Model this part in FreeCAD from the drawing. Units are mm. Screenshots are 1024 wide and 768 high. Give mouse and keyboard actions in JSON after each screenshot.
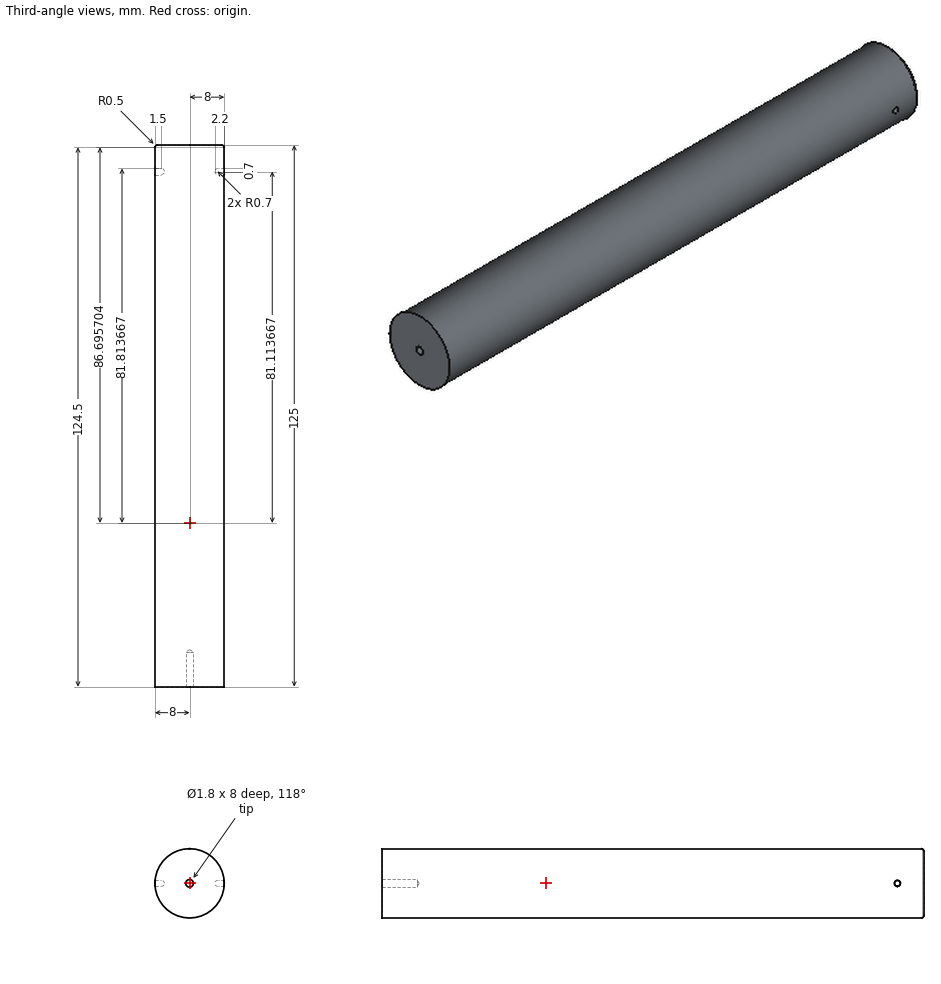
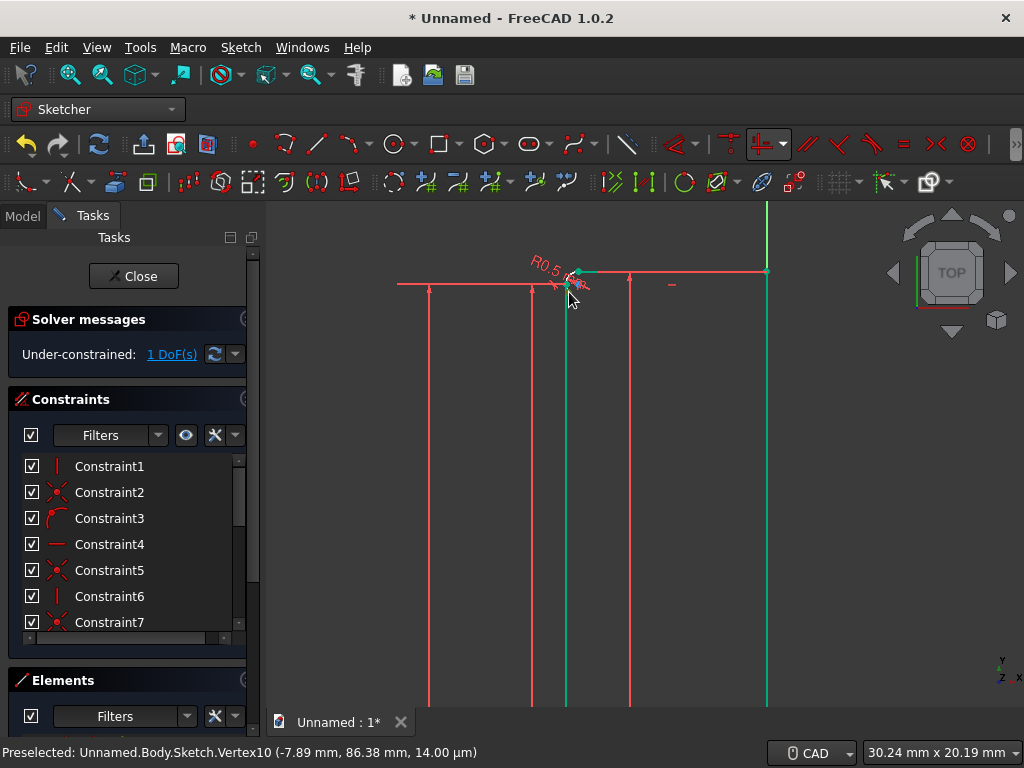
{"action": "key", "text": "i"}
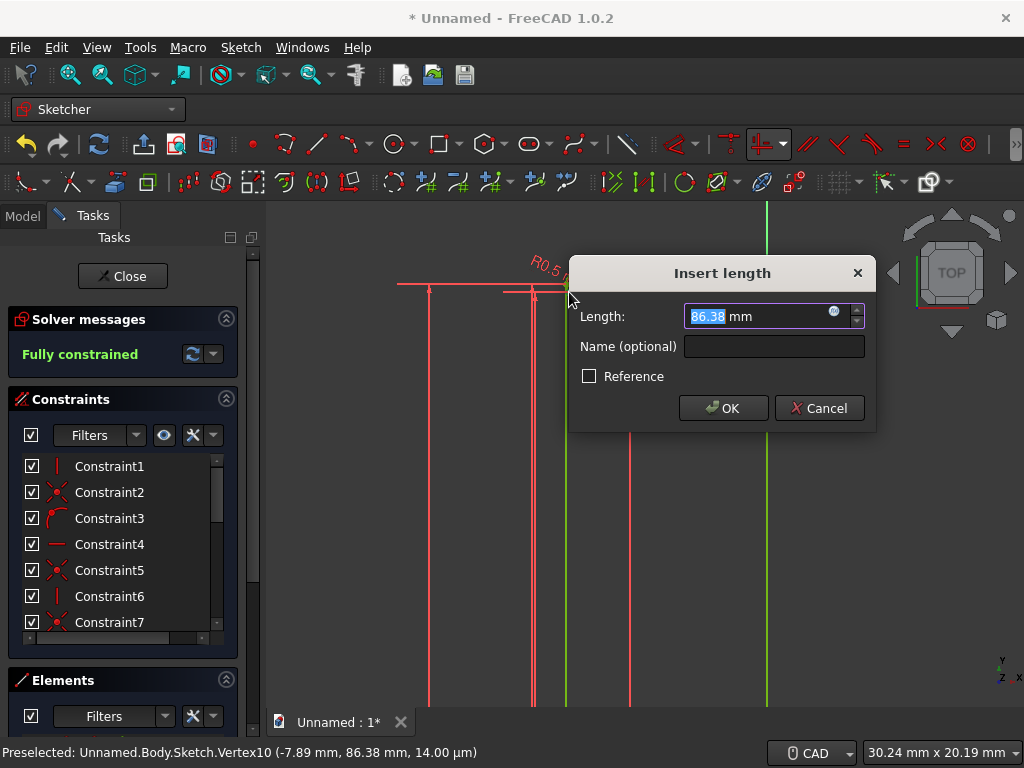
{"action": "type", "text": "86.695704"}
{"action": "key", "text": "Return"}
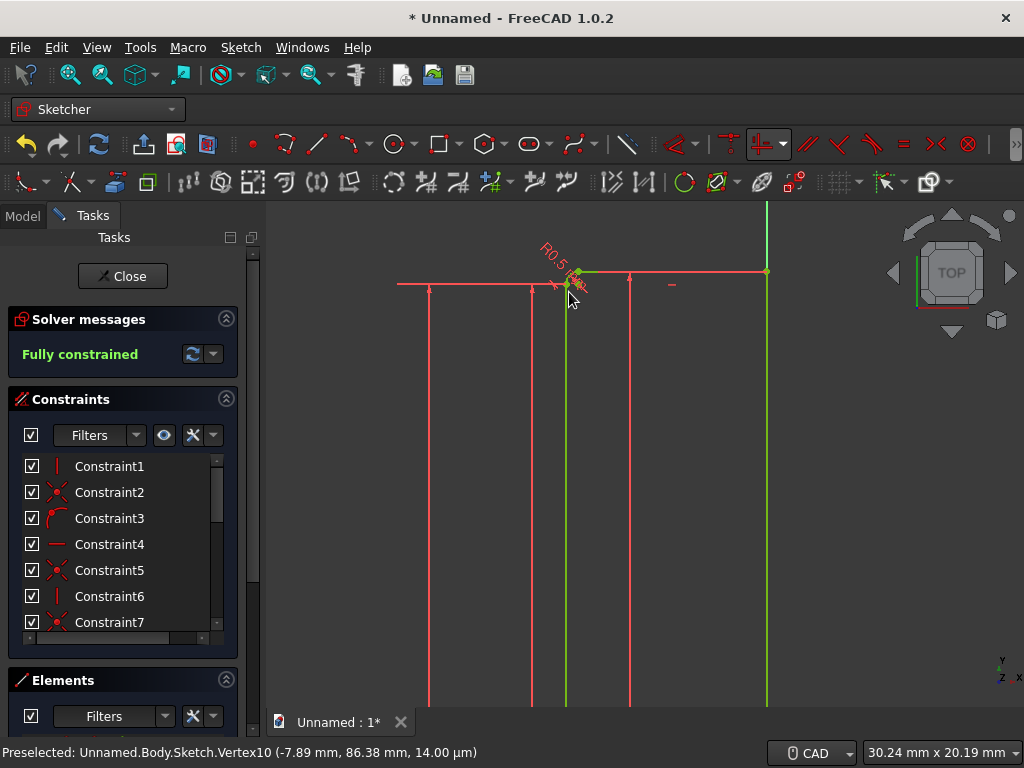
{"action": "left_click", "coordinate": [123, 276]}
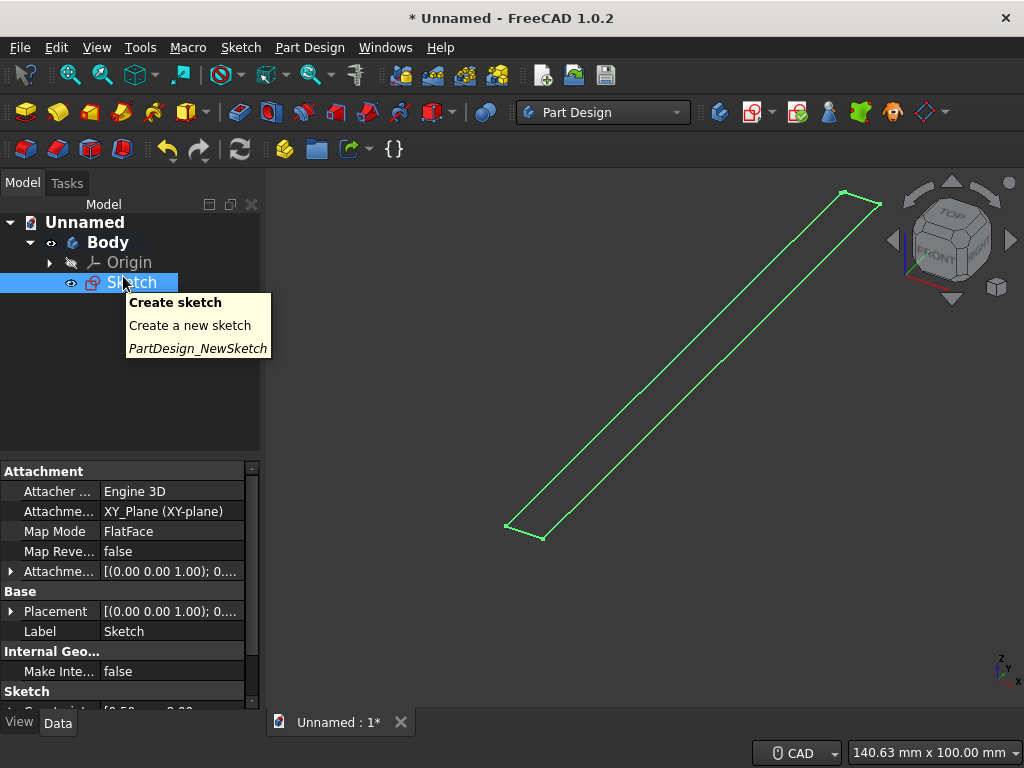
{"action": "left_click", "coordinate": [58, 112]}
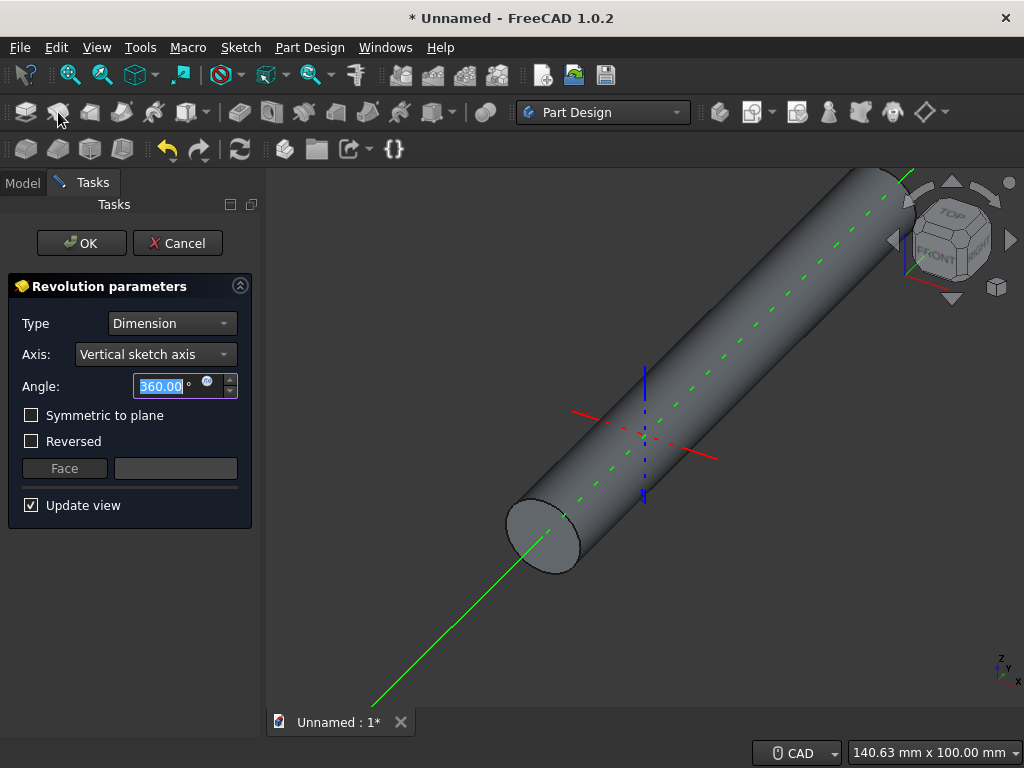
{"action": "left_click", "coordinate": [82, 243]}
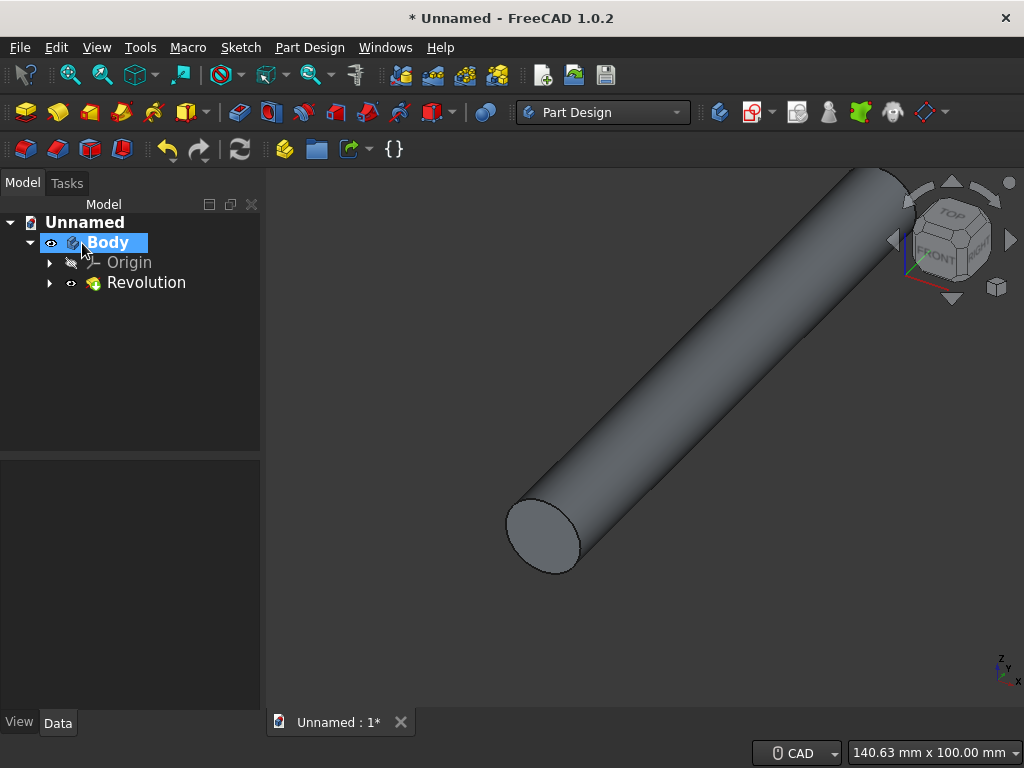
{"action": "left_click", "coordinate": [72, 76]}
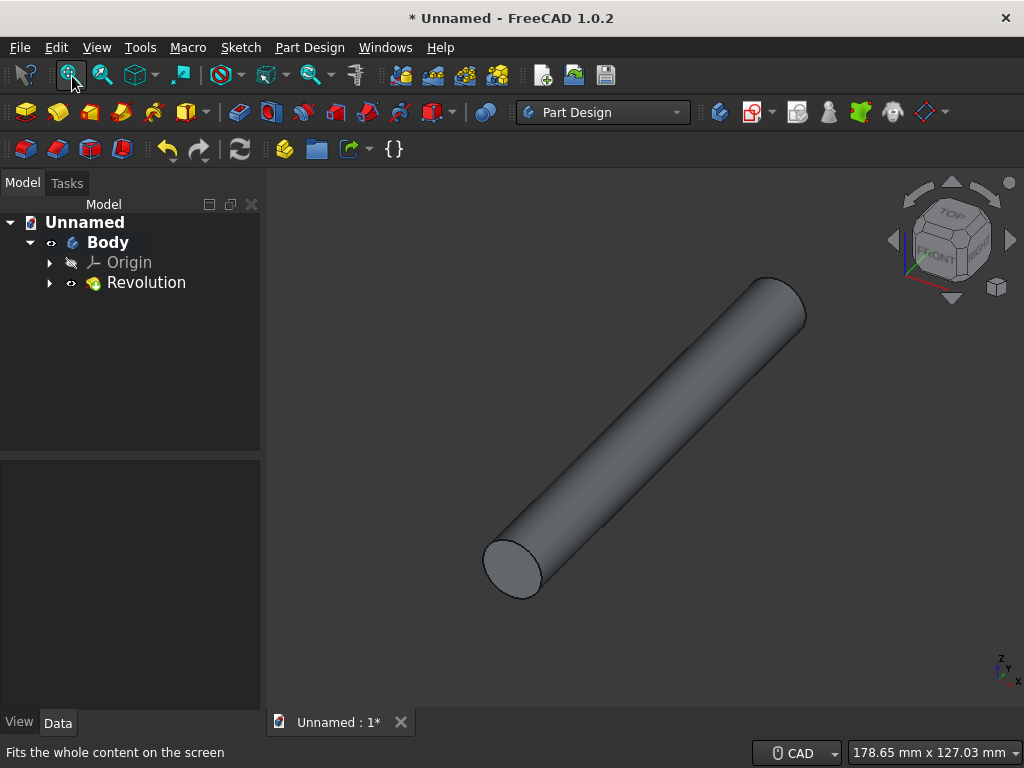
{"action": "left_click", "coordinate": [752, 112]}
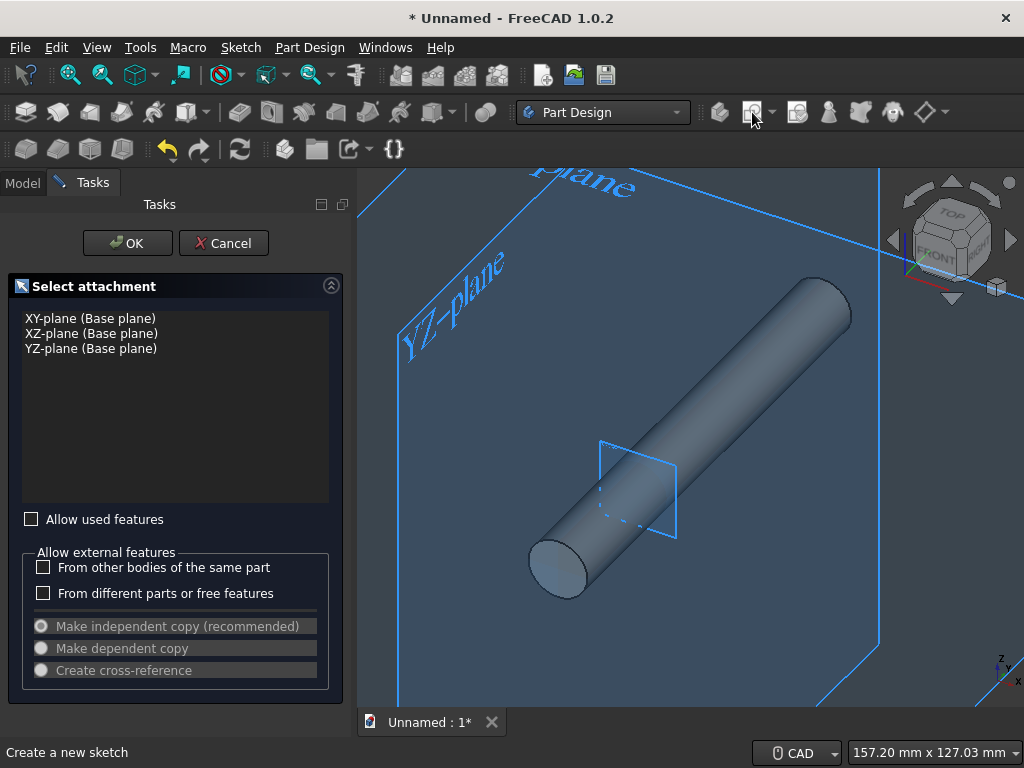
{"action": "left_click", "coordinate": [82, 318]}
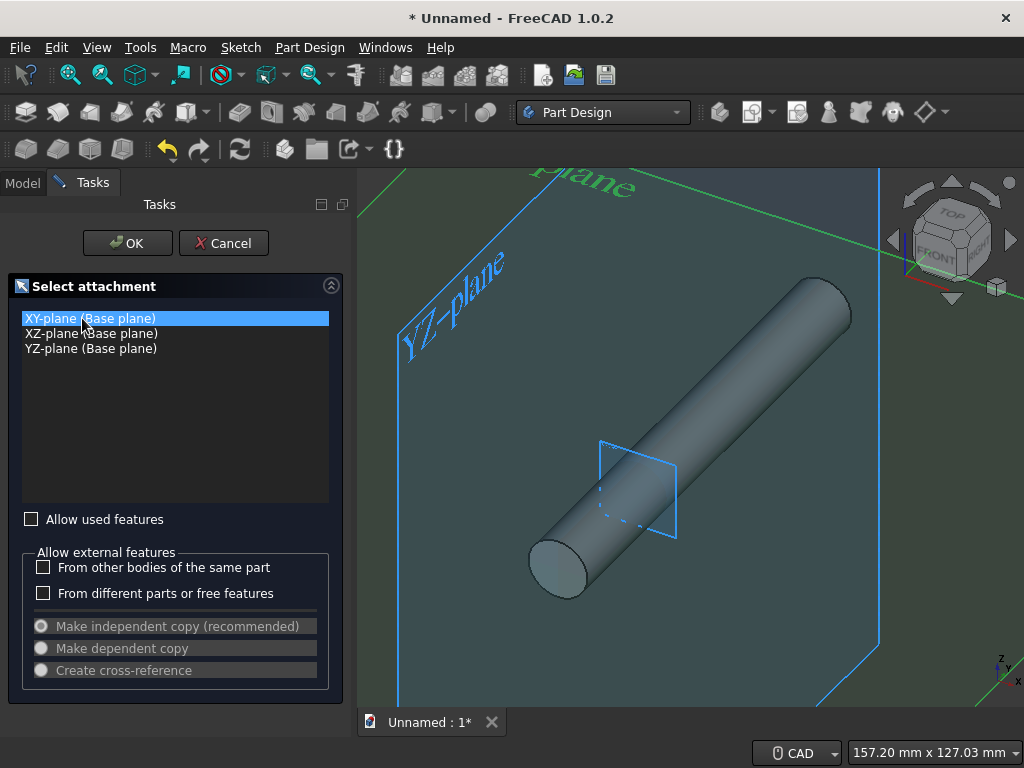
{"action": "left_click", "coordinate": [128, 243]}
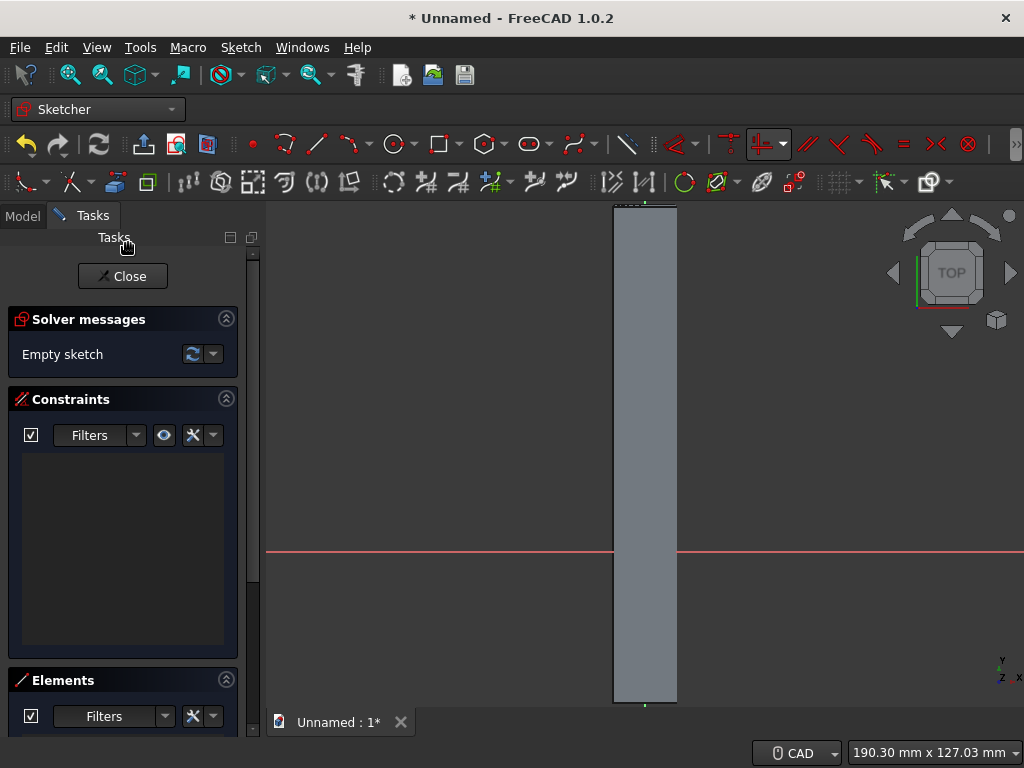
{"action": "key", "text": "q s"}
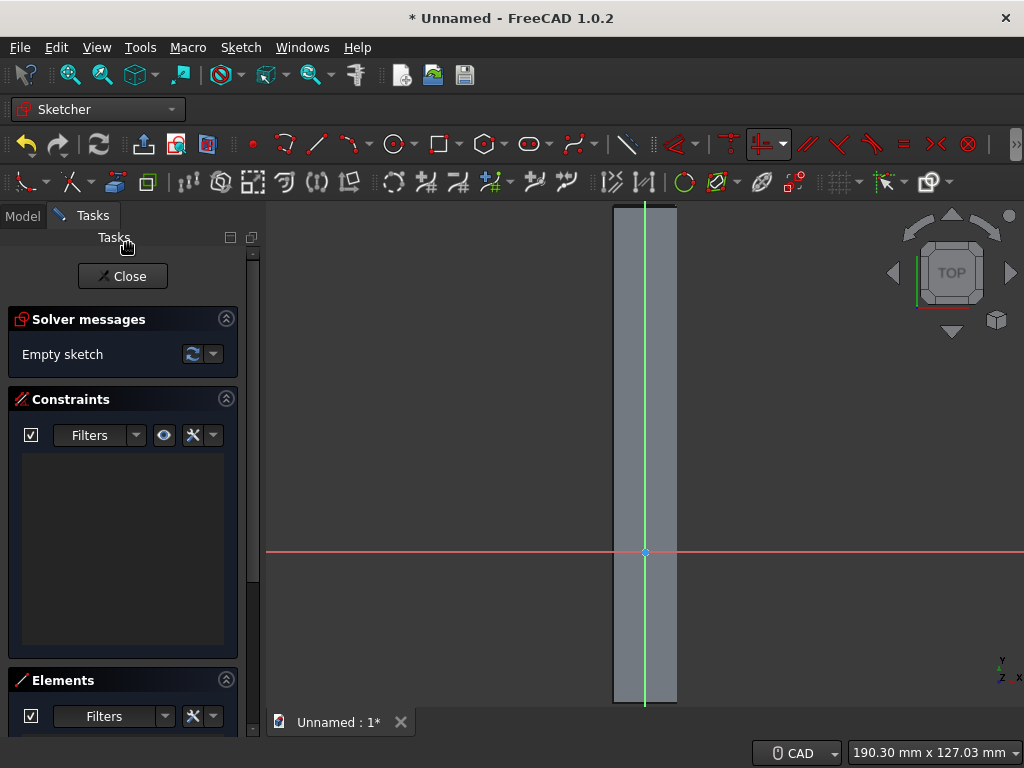
{"action": "scroll", "coordinate": [576, 454], "scroll_direction": "down", "scroll_amount": 5}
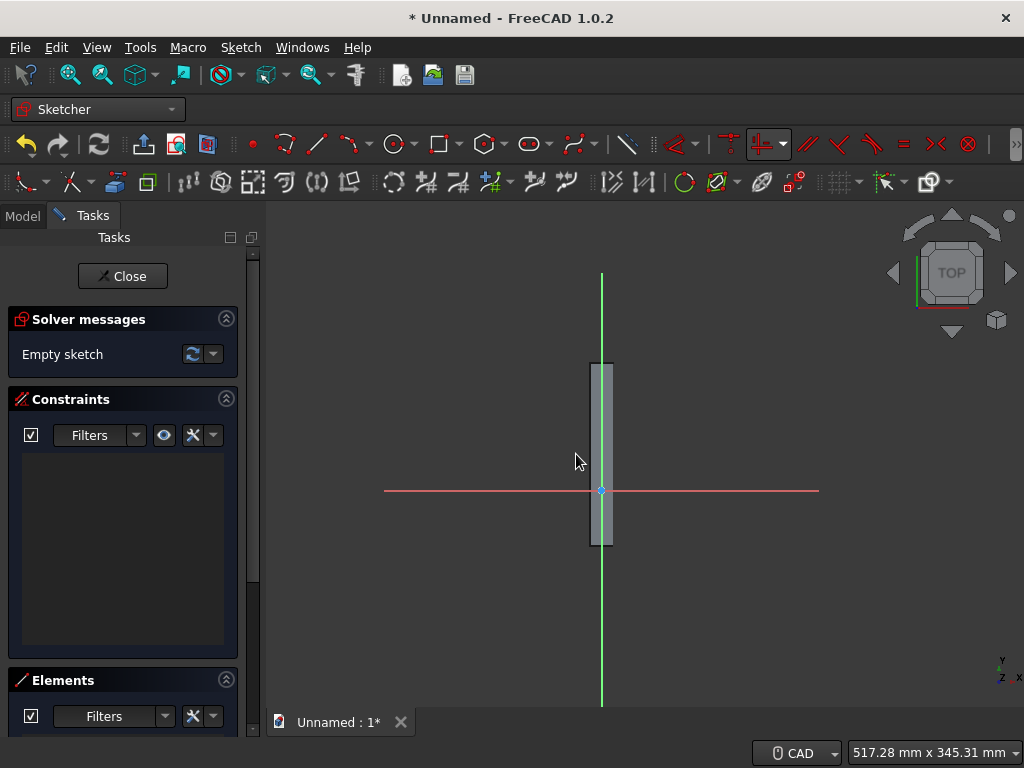
{"action": "scroll", "coordinate": [599, 363], "scroll_direction": "up", "scroll_amount": 12}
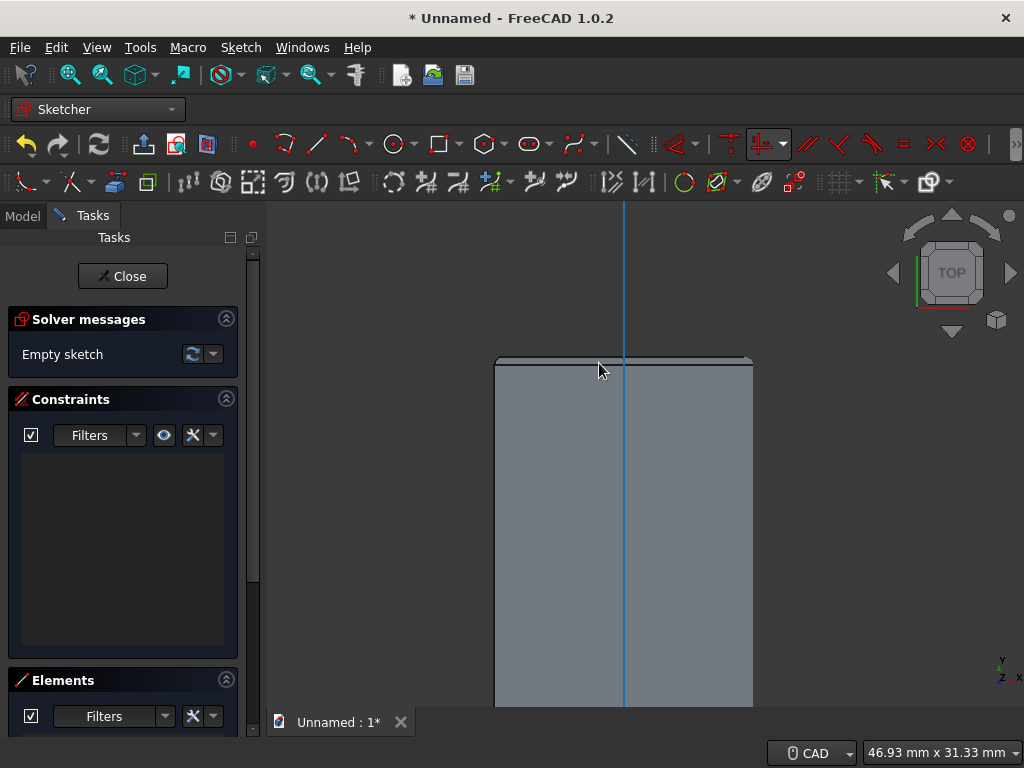
{"action": "key", "text": "g m"}